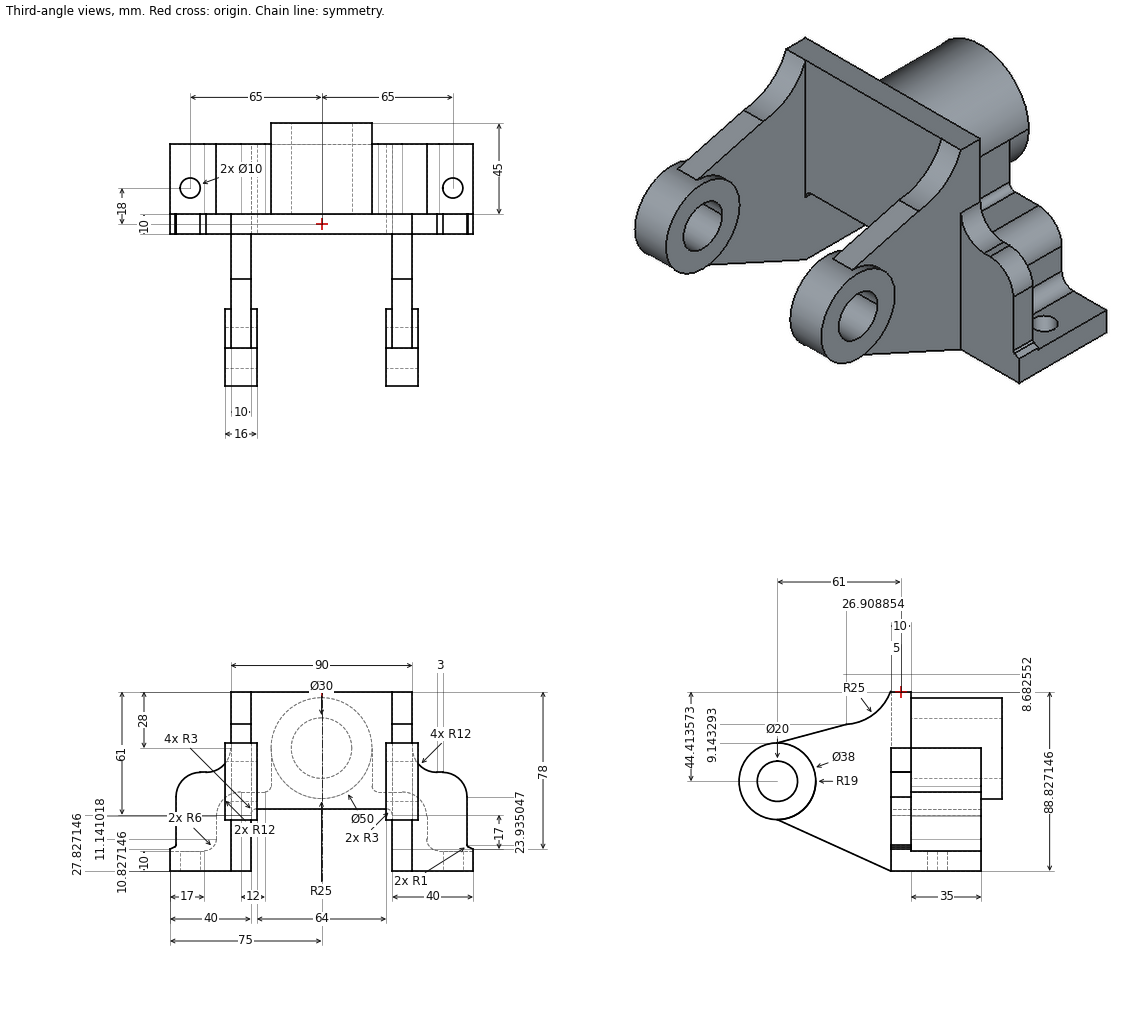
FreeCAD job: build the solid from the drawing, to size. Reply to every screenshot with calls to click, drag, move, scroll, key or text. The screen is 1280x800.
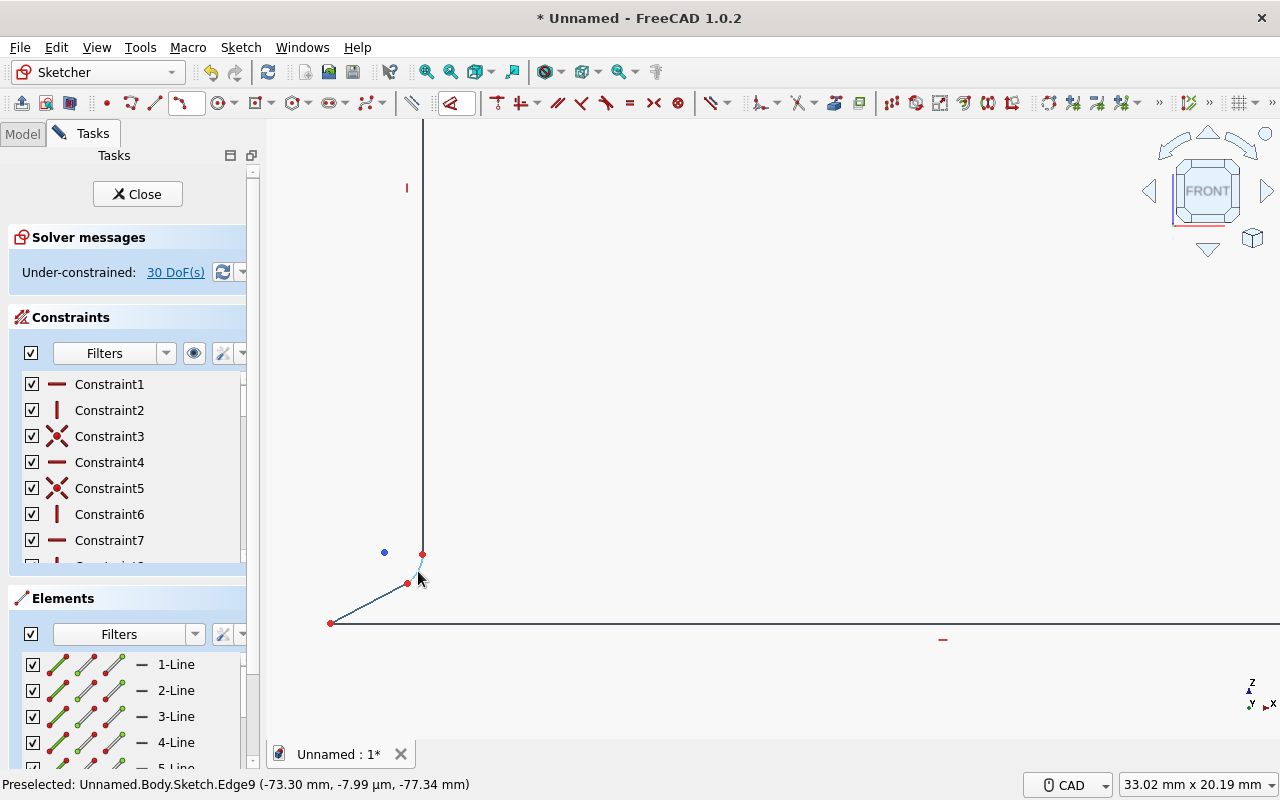
click(418, 571)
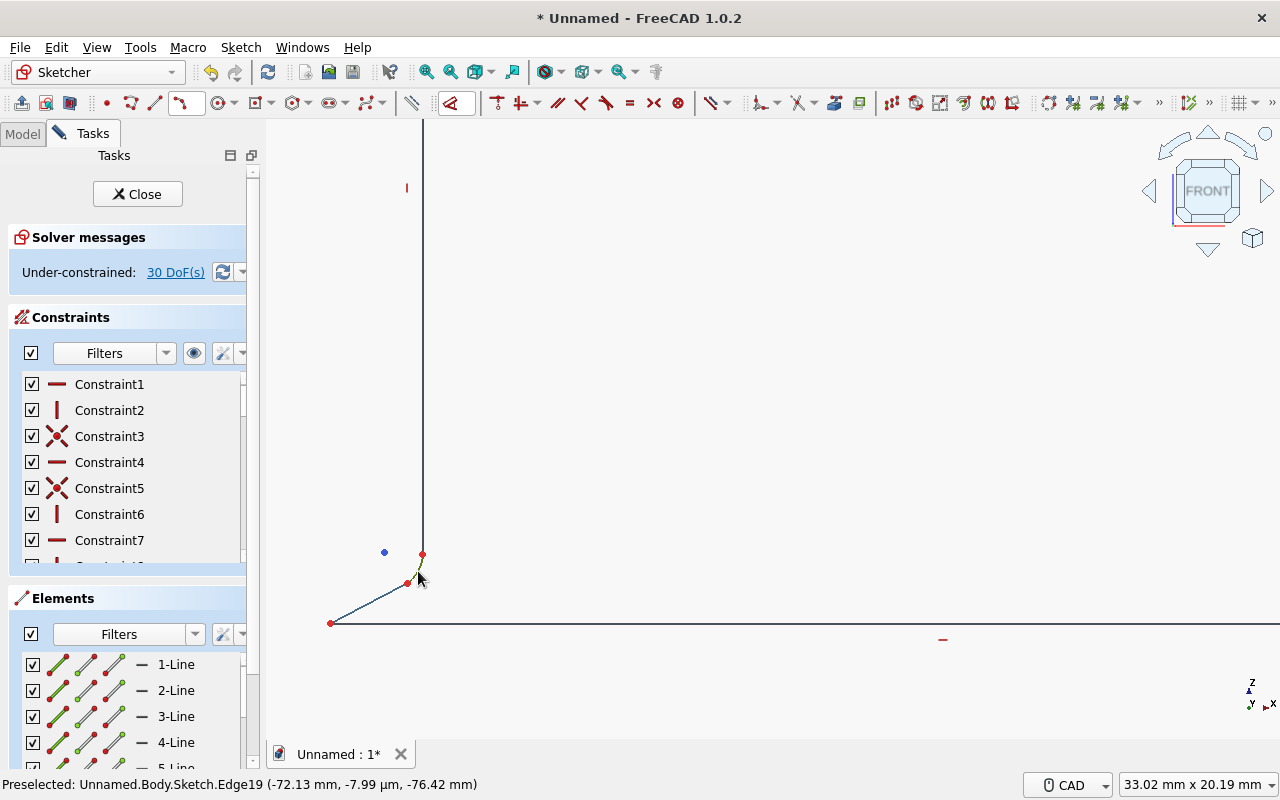
click(606, 104)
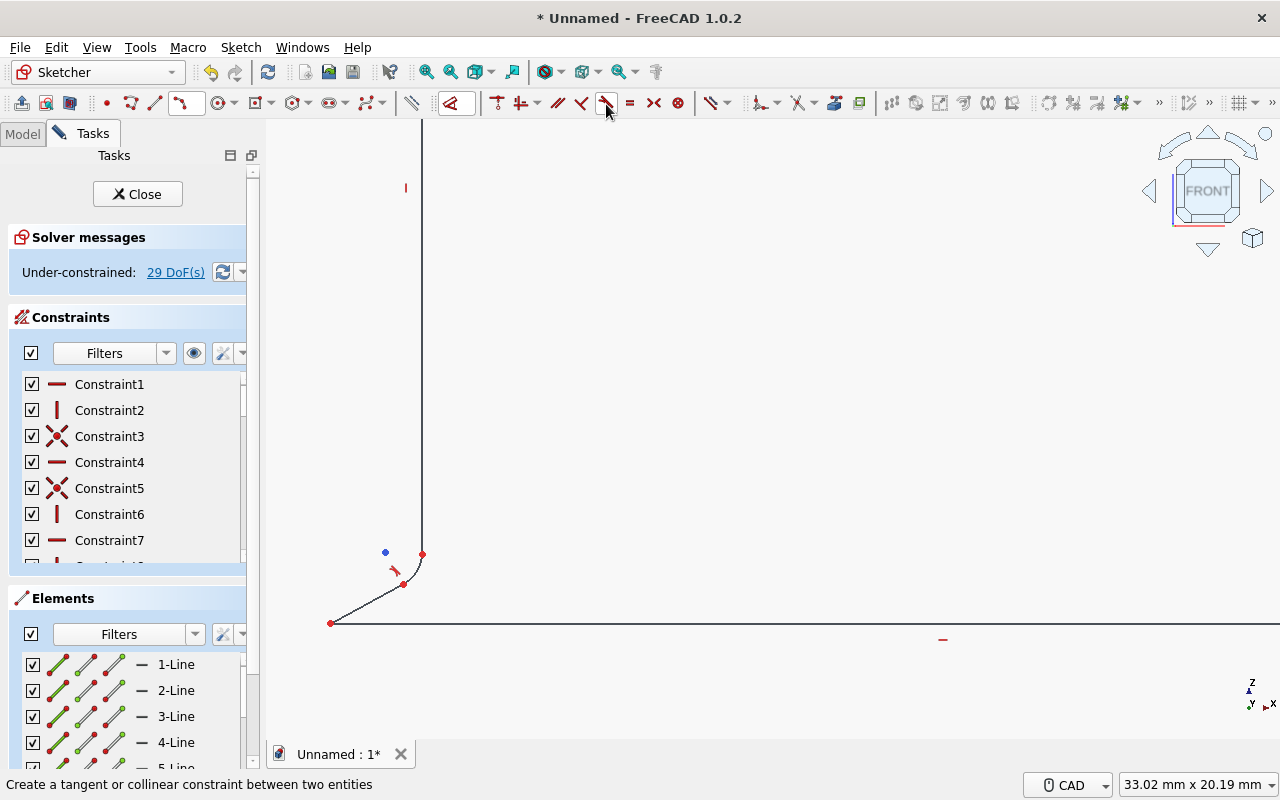
scroll(402, 587, down, 10)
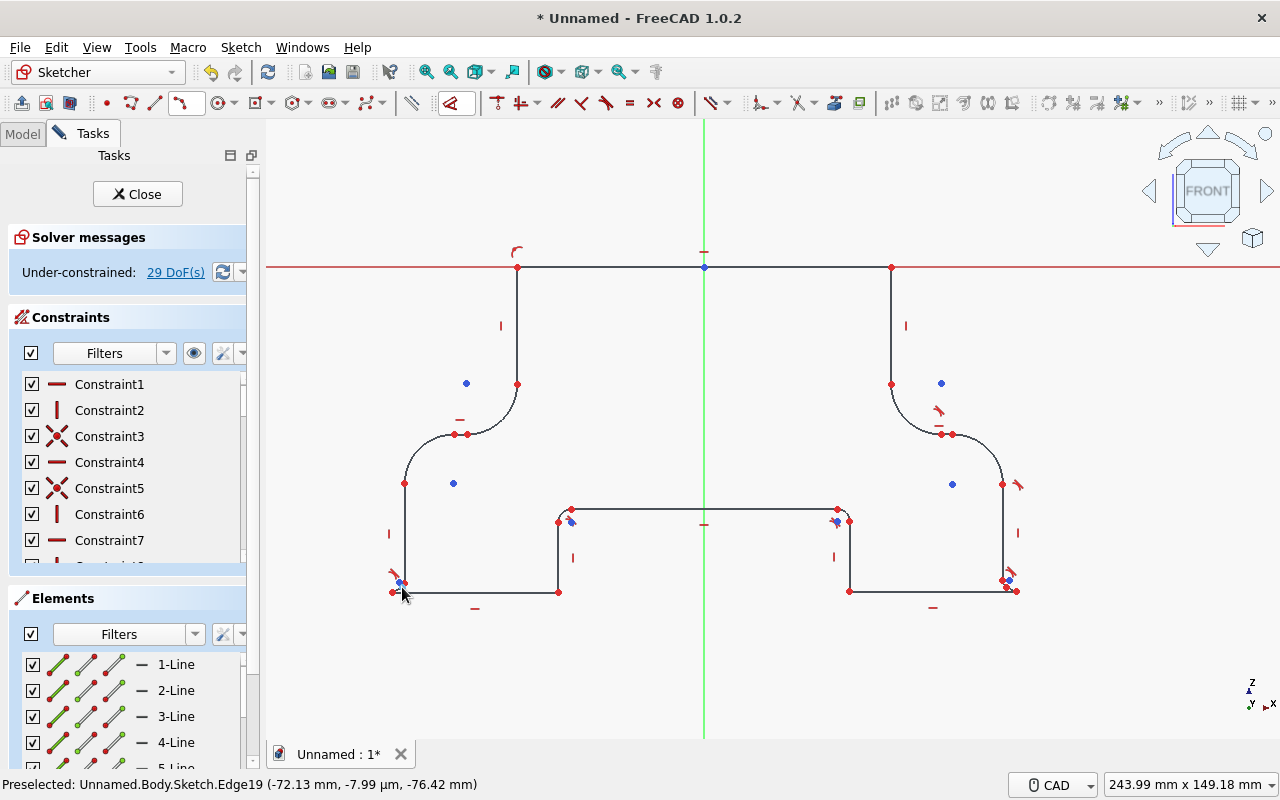
click(405, 553)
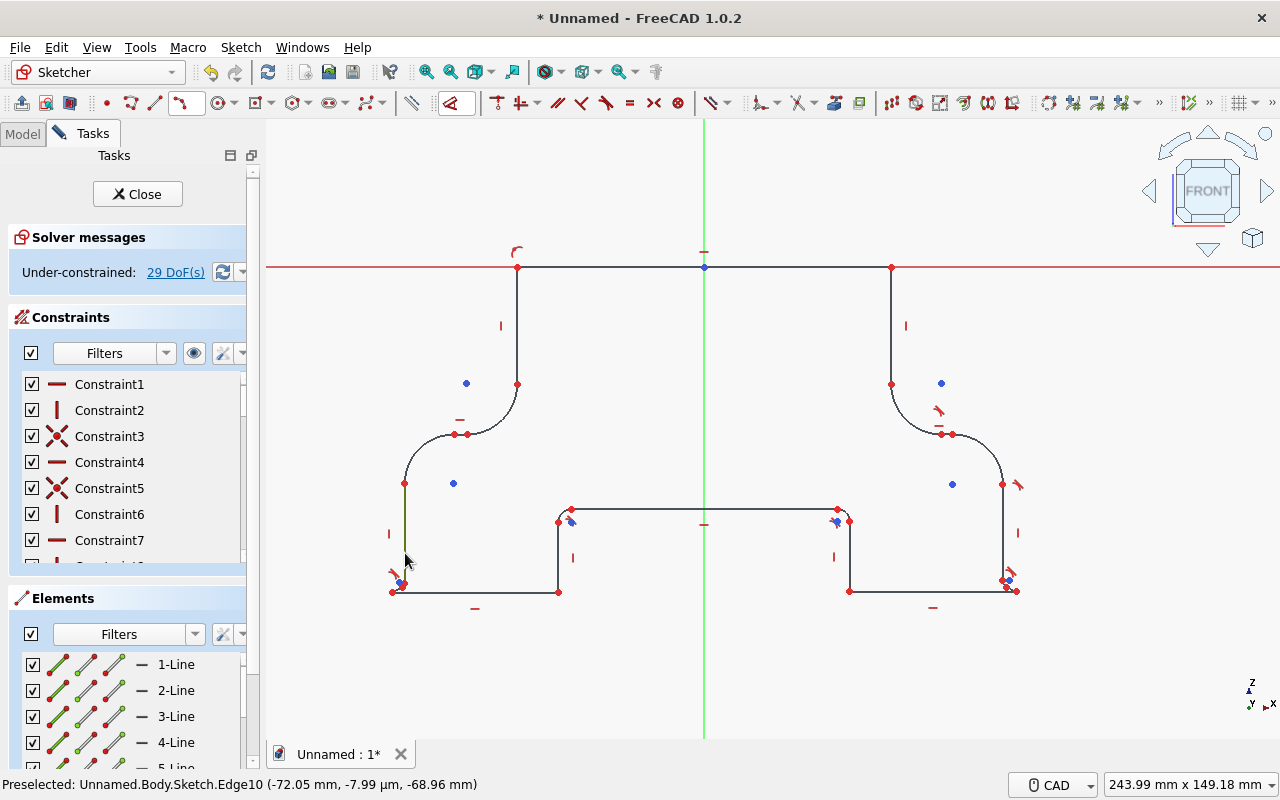
scroll(404, 586, up, 9)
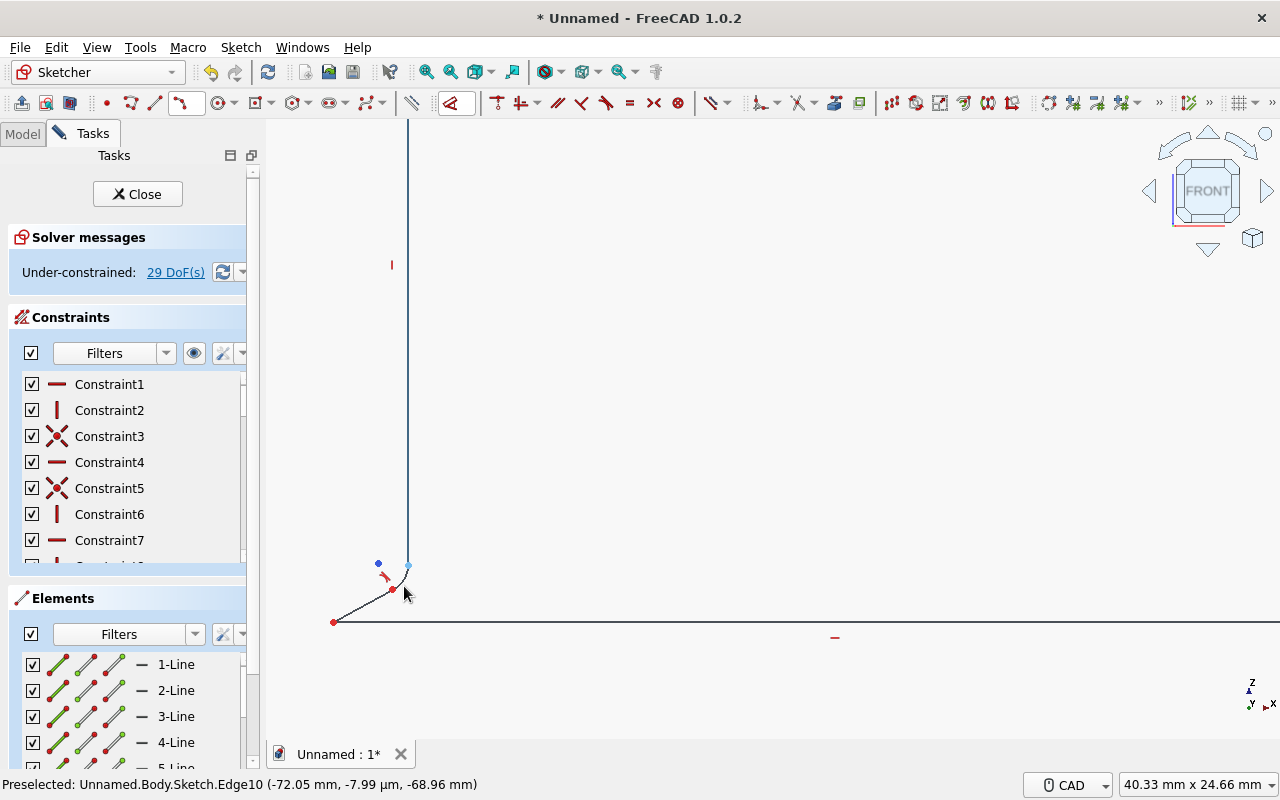
click(404, 580)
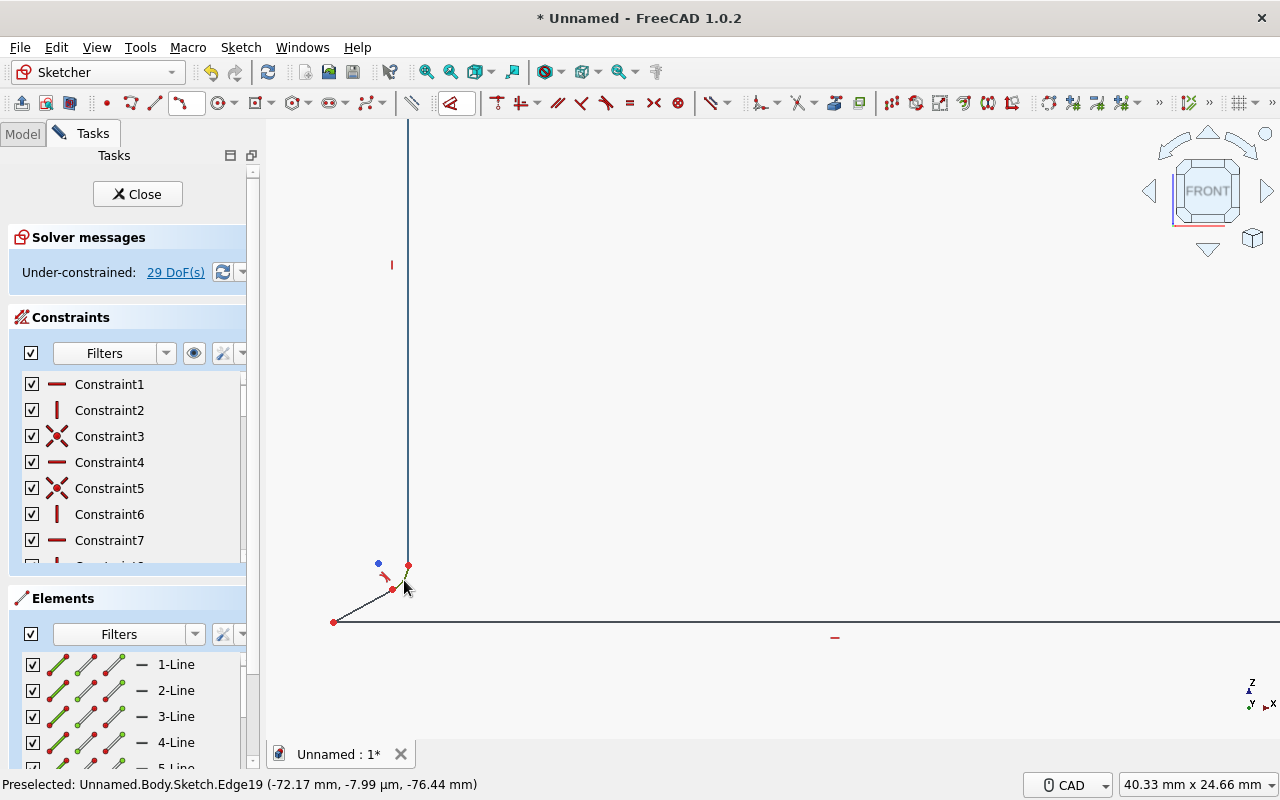
key(t)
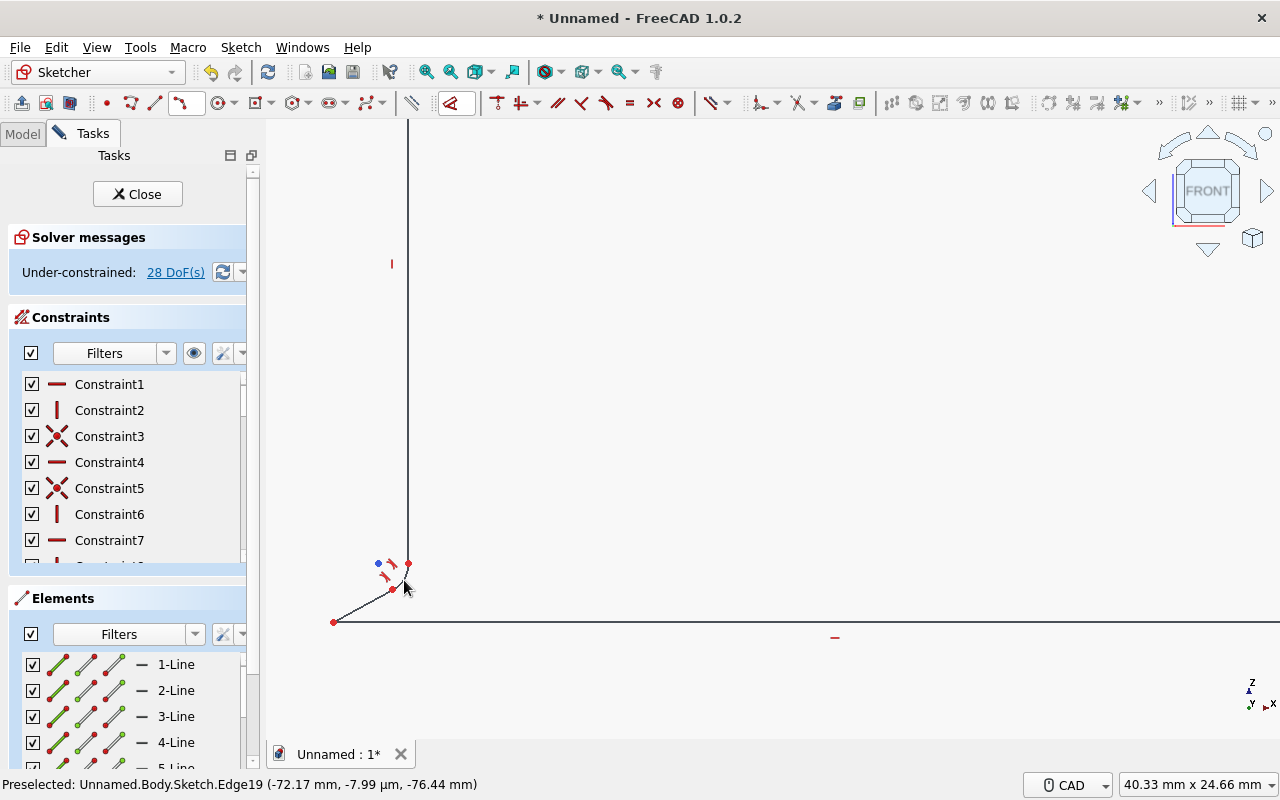
scroll(404, 586, down, 9)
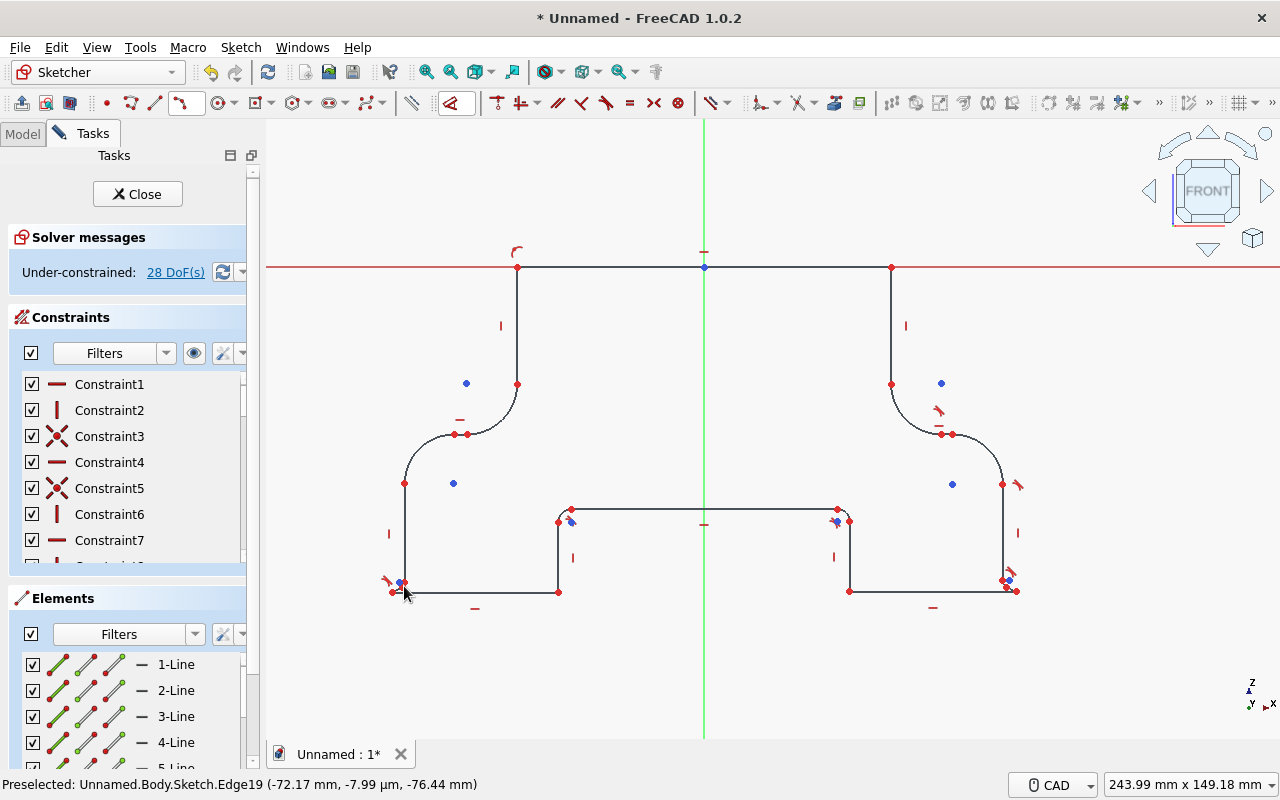
click(405, 553)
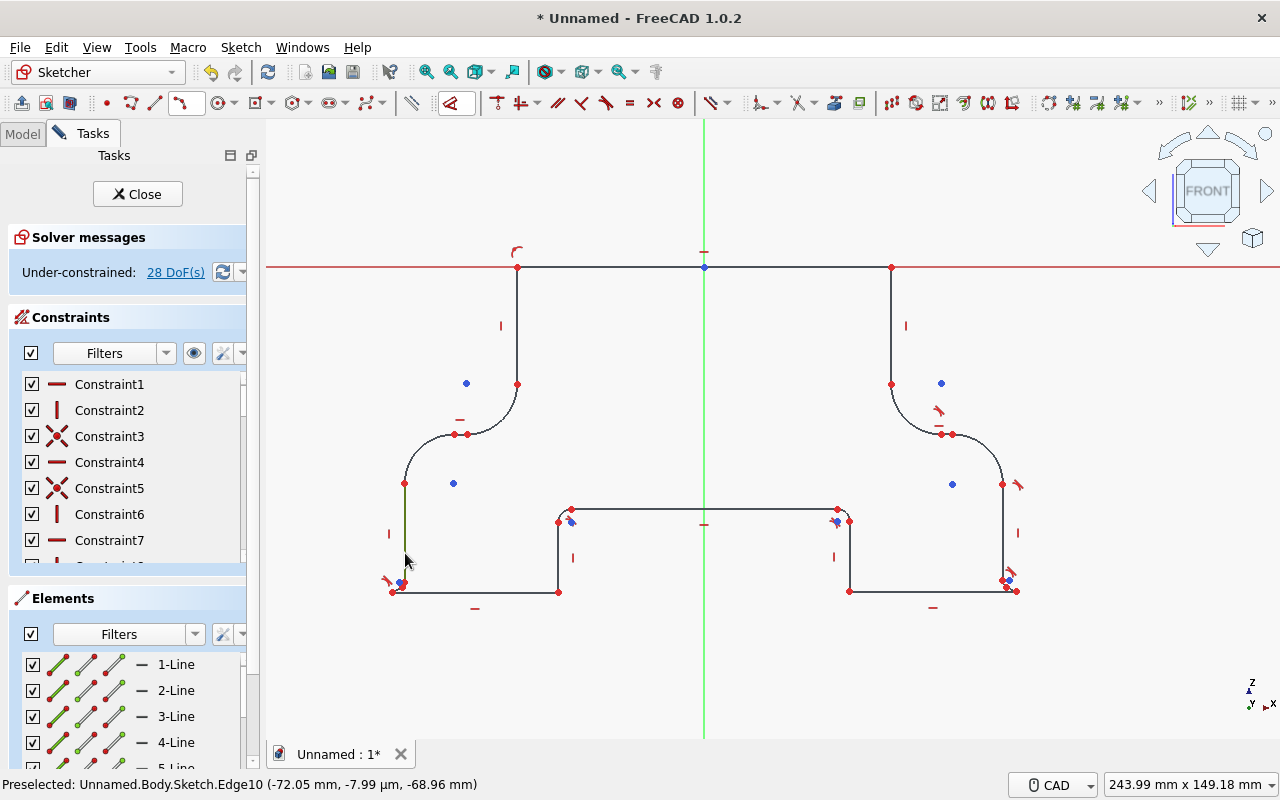
click(432, 440)